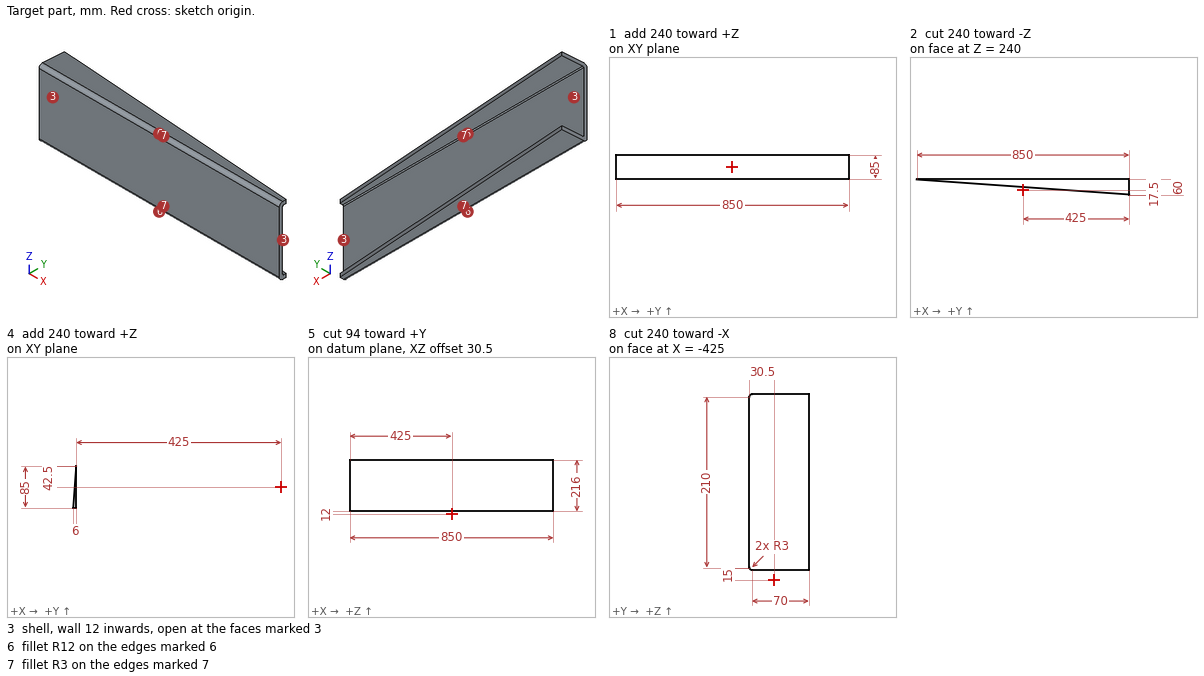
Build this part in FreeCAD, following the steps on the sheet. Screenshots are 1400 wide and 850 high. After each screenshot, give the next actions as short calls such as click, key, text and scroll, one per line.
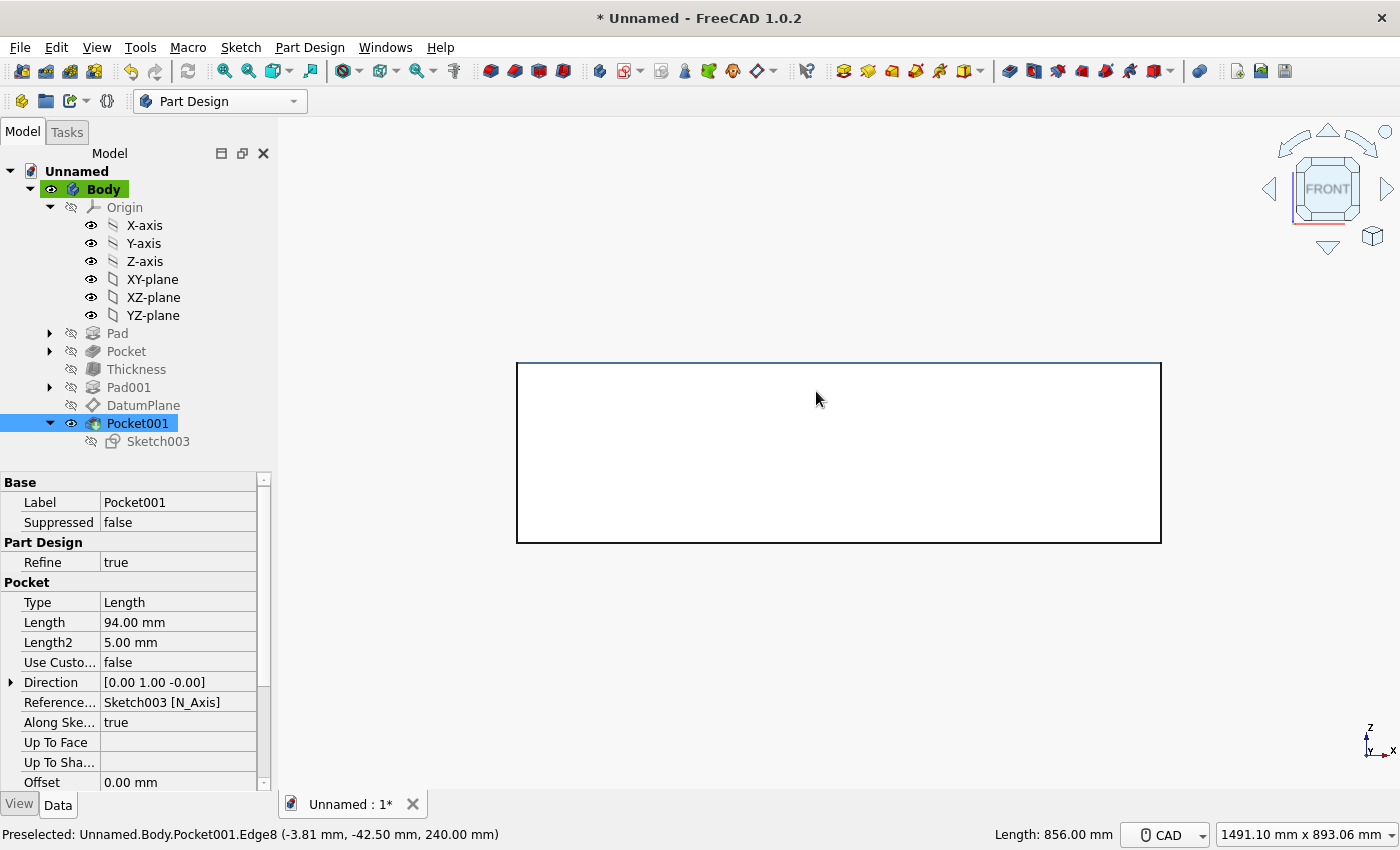
click(839, 542, ctrl)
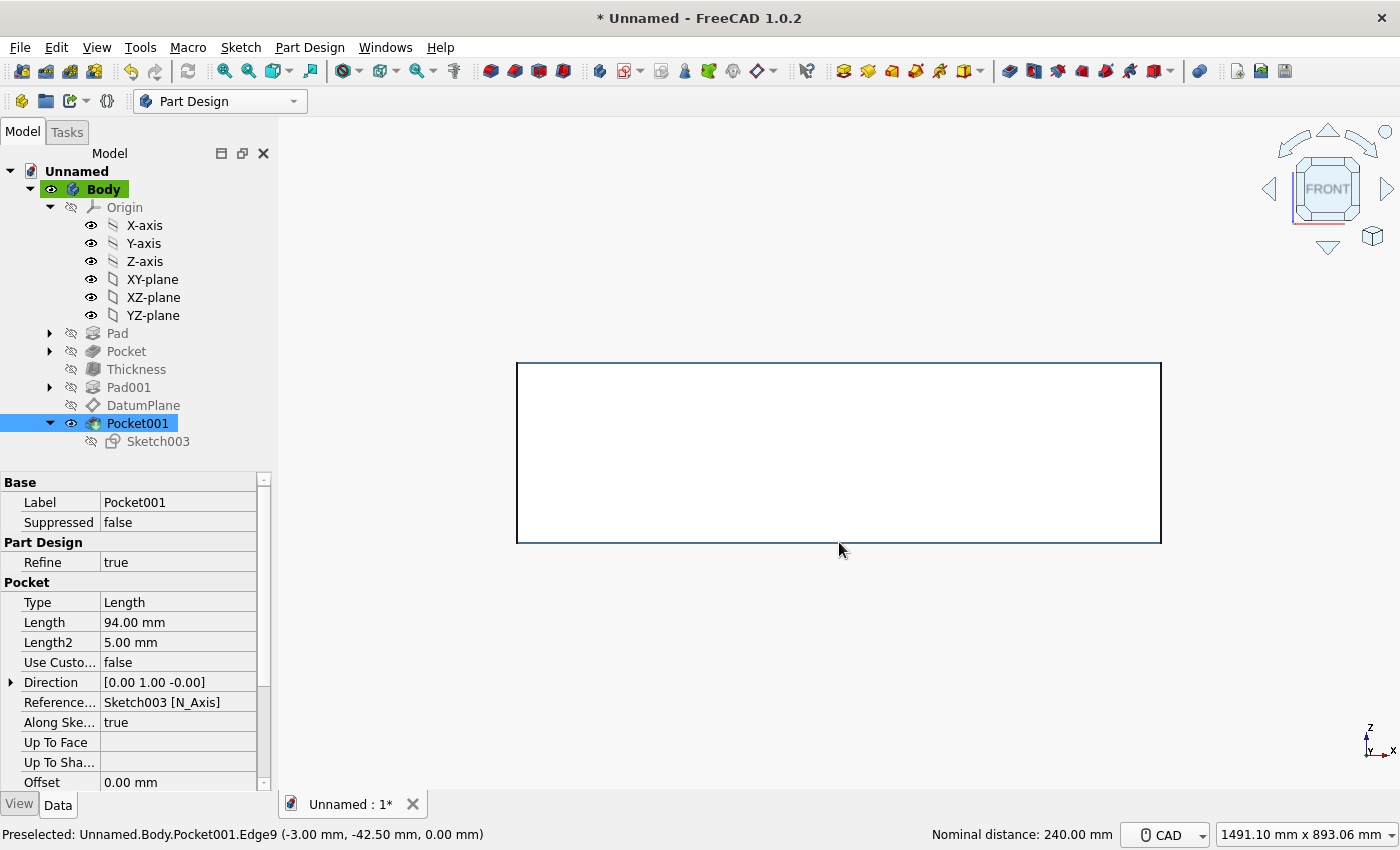
click(492, 72)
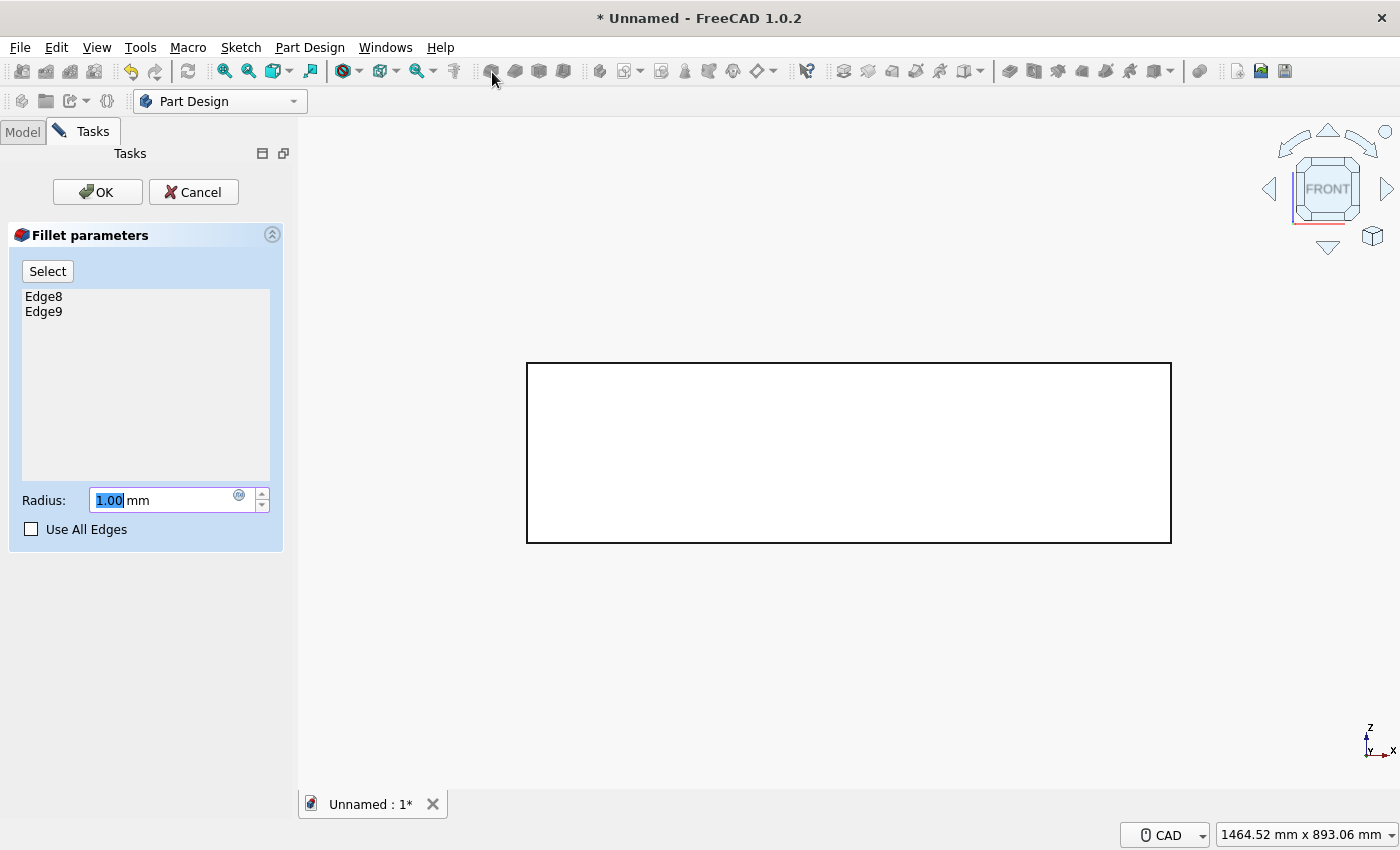
text(12)
key(Tab)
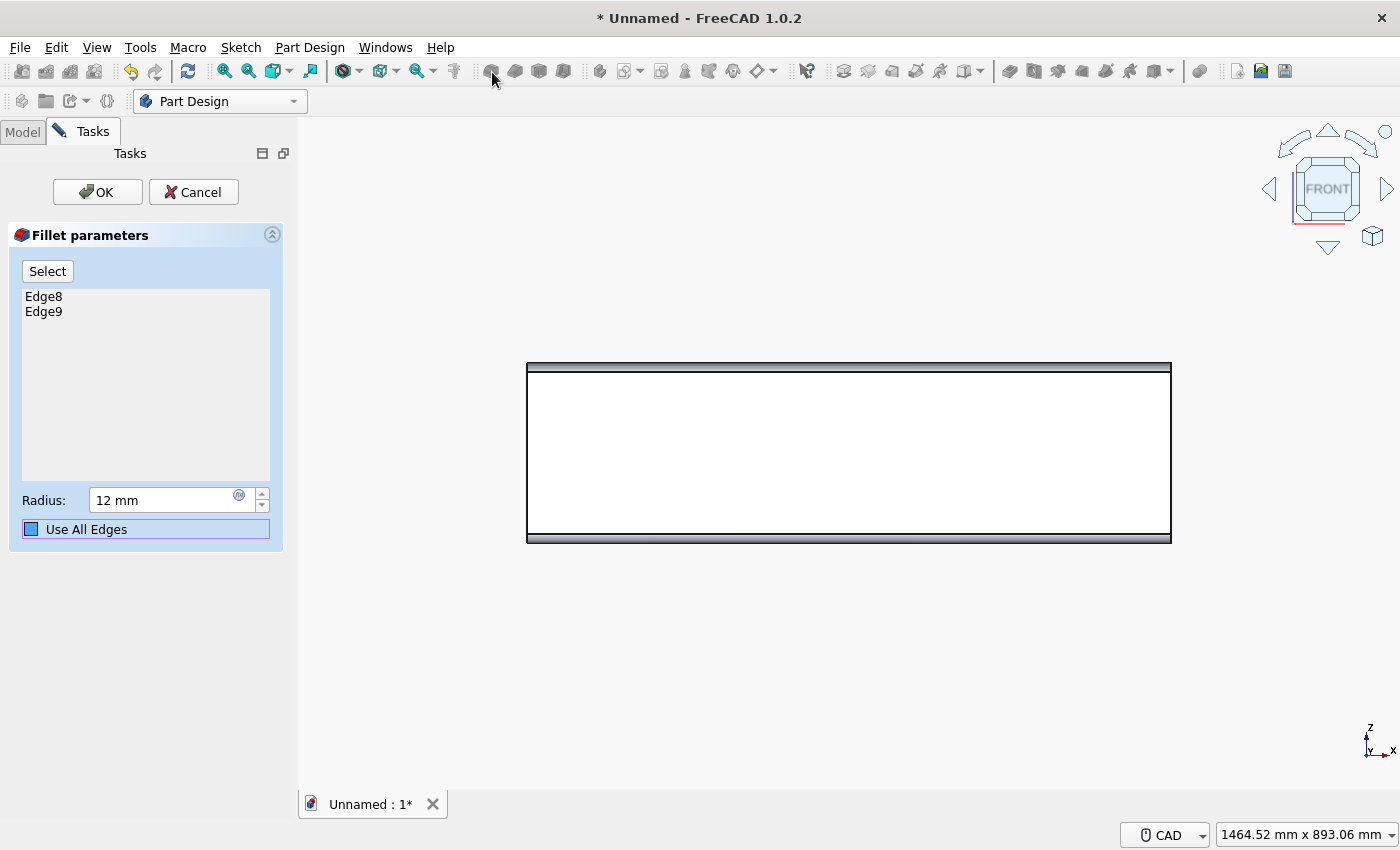
click(98, 192)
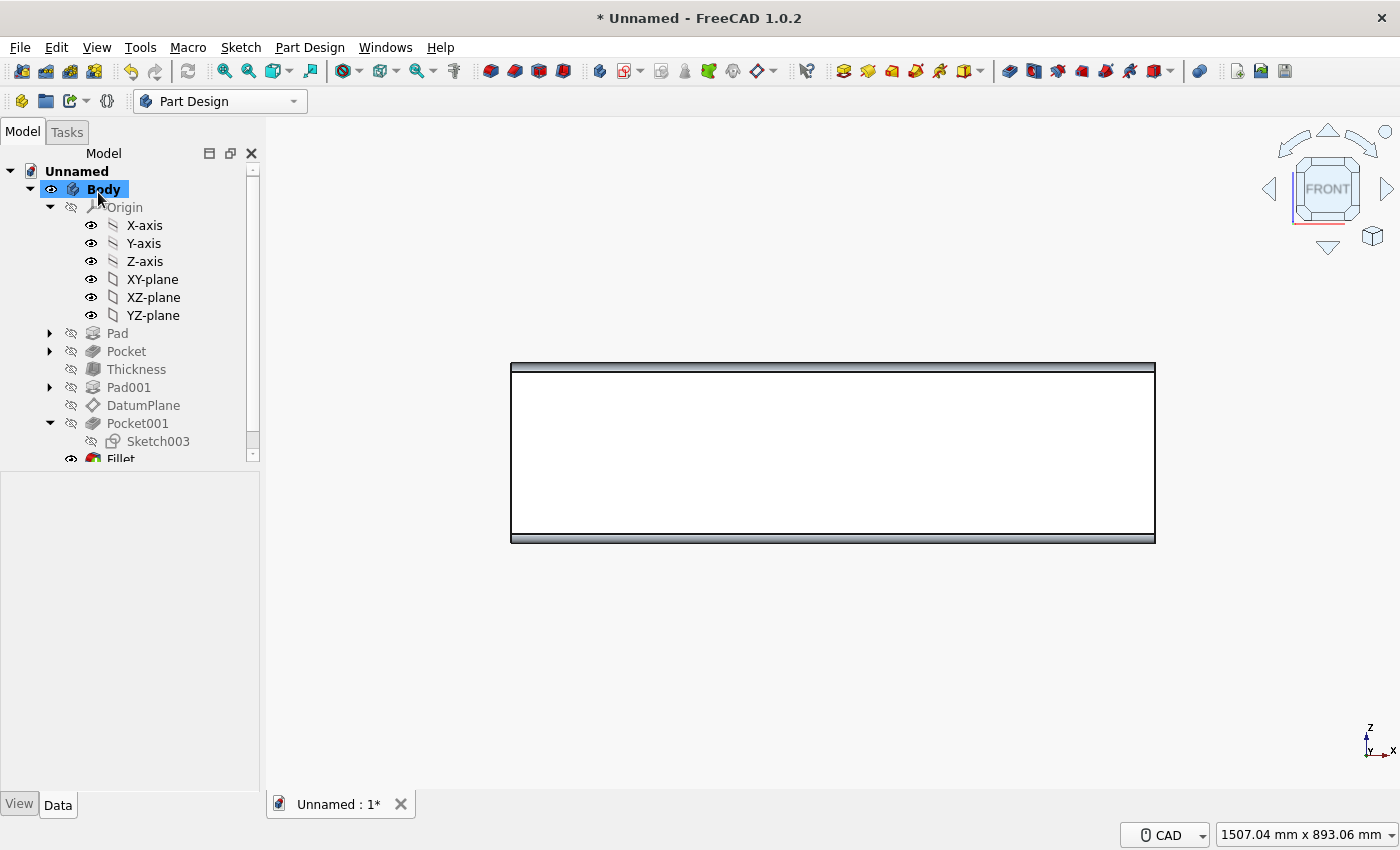
key(0)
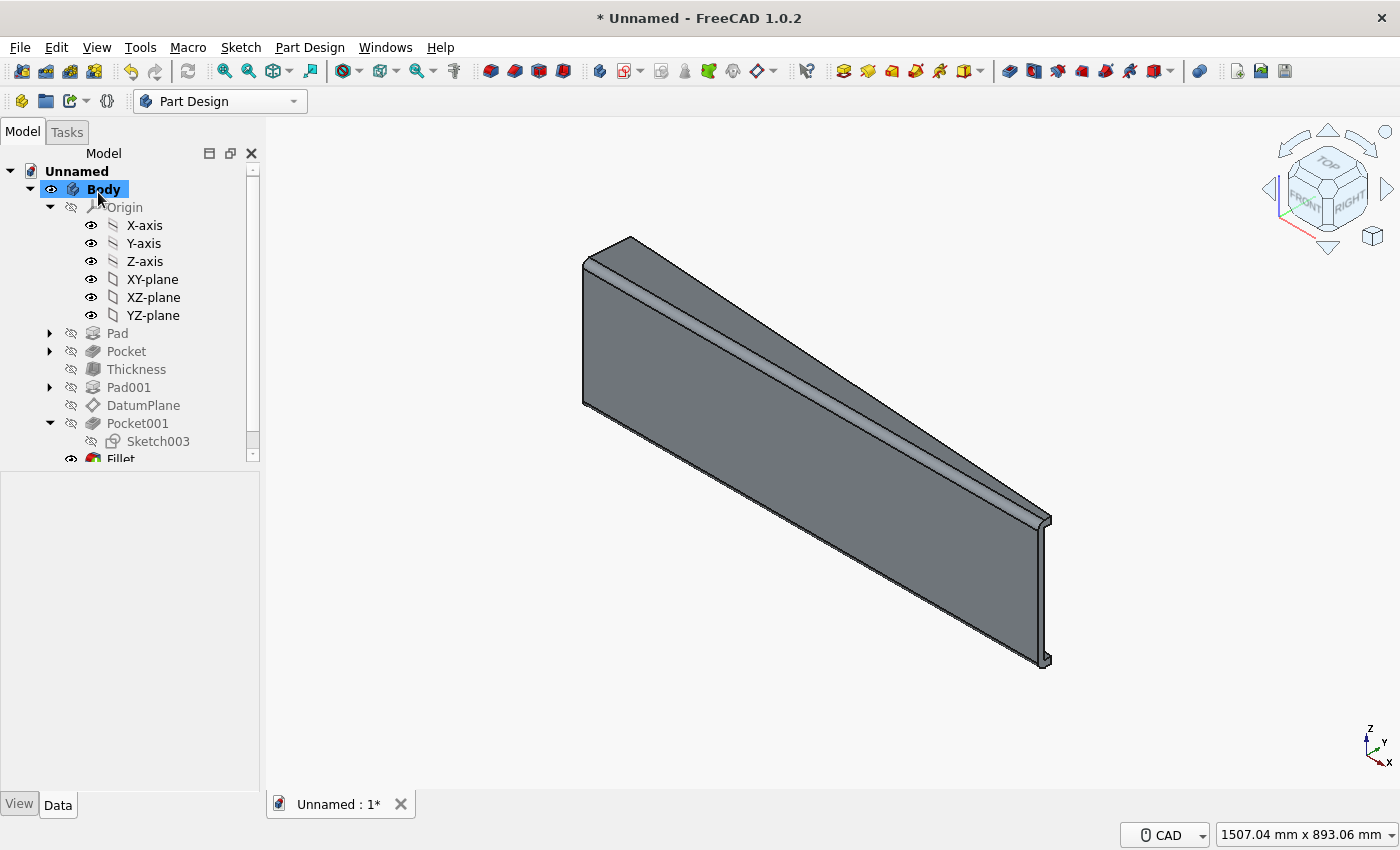
key(2)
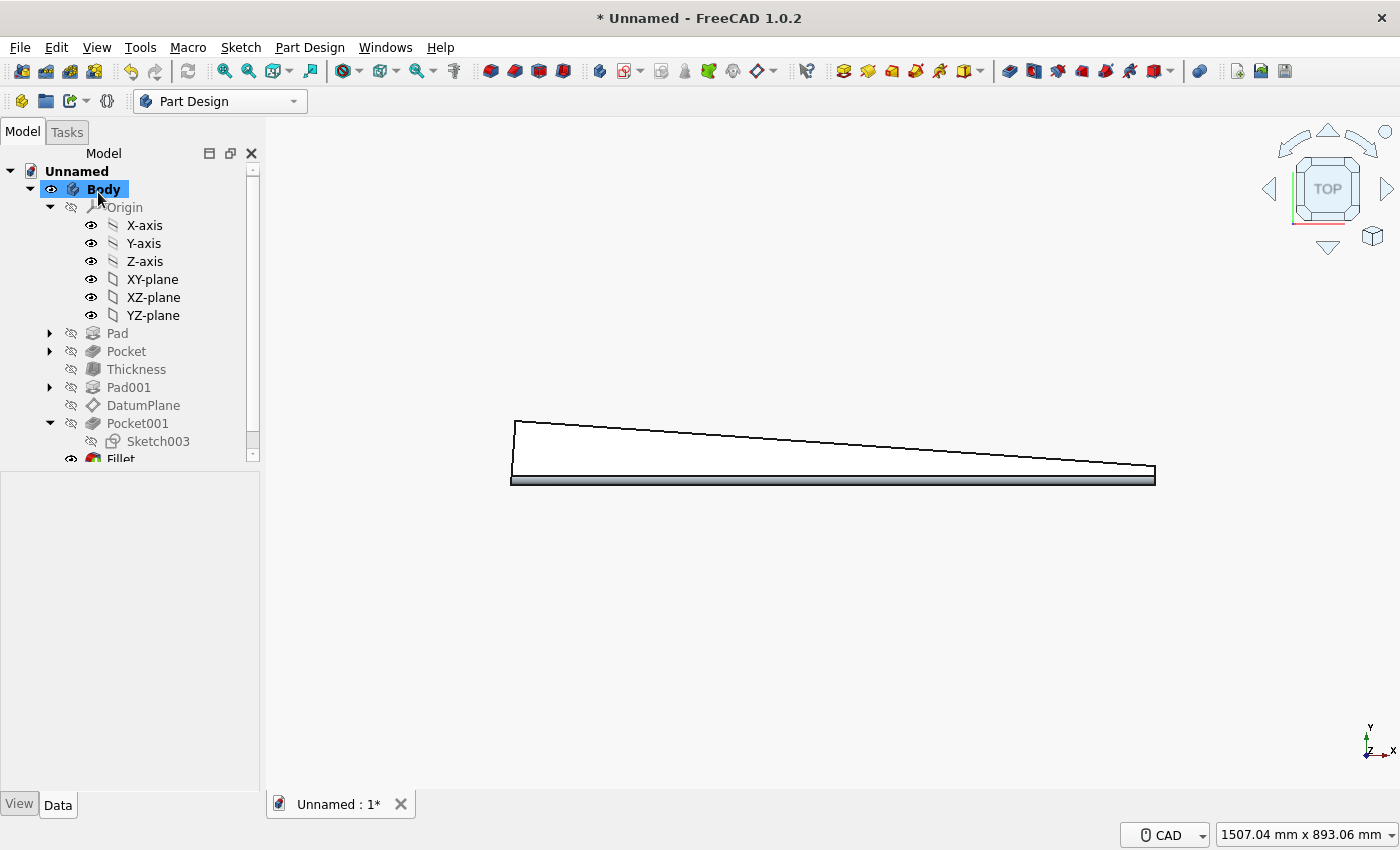
key(1)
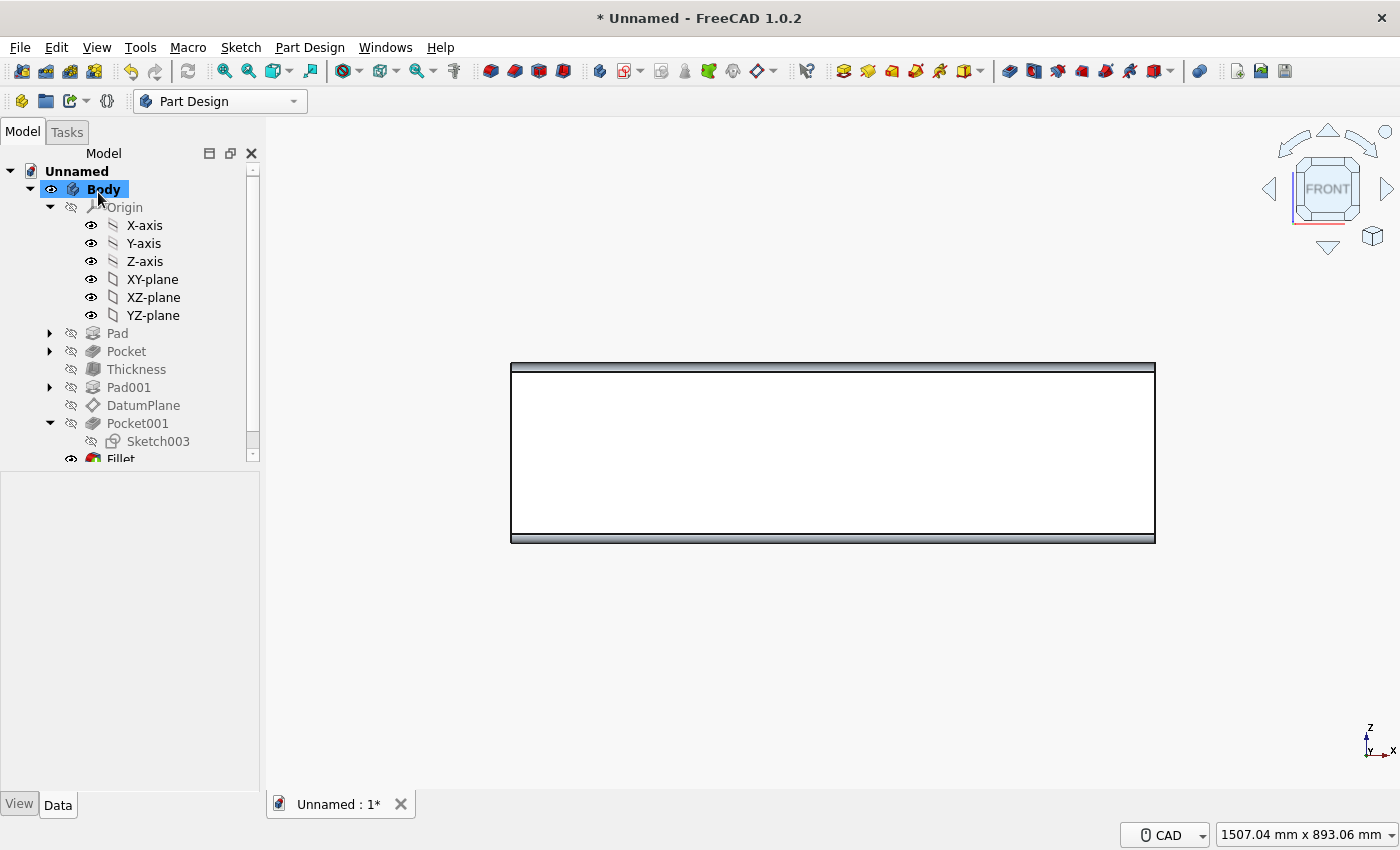
key(3)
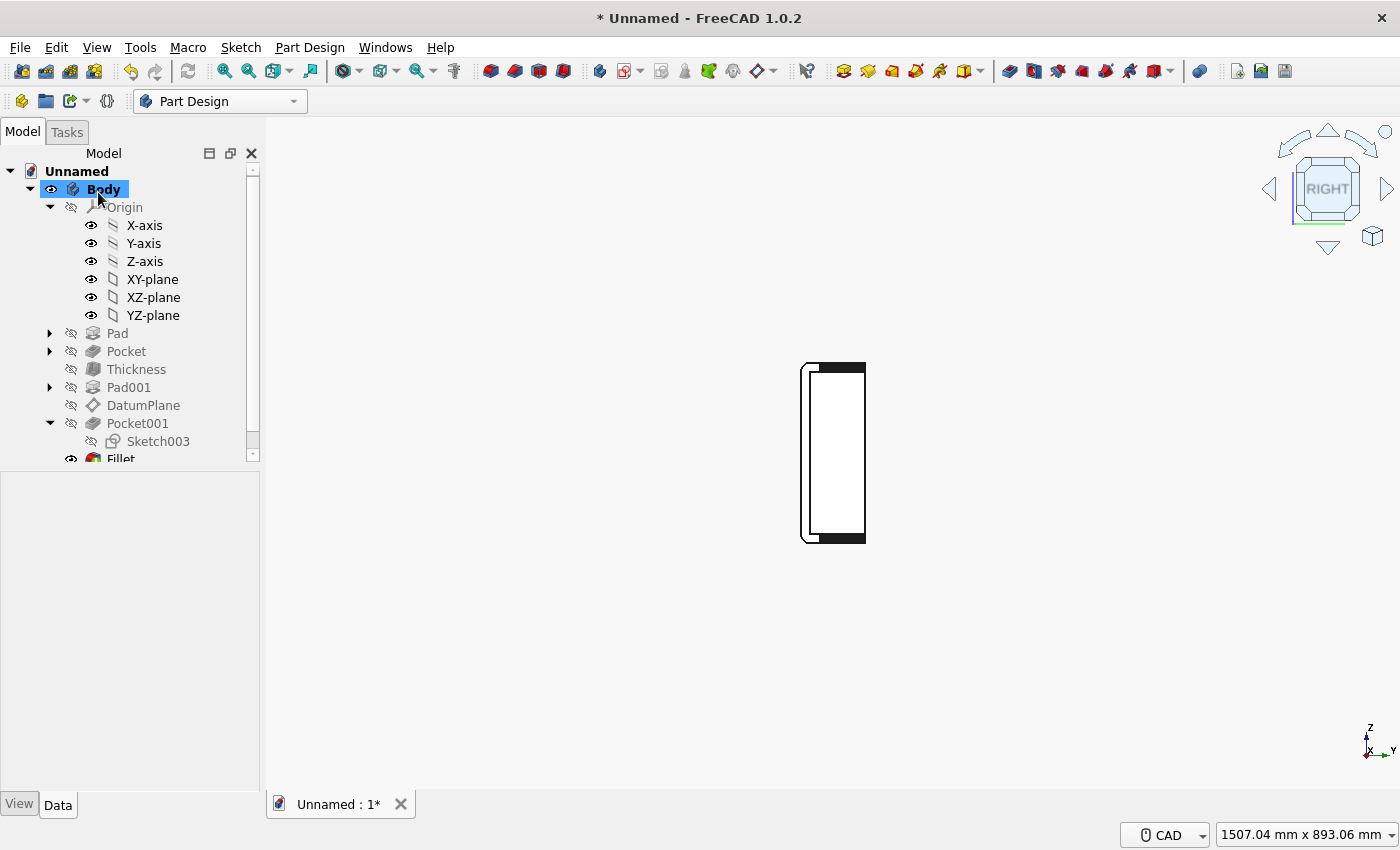
key(v)
key(f)